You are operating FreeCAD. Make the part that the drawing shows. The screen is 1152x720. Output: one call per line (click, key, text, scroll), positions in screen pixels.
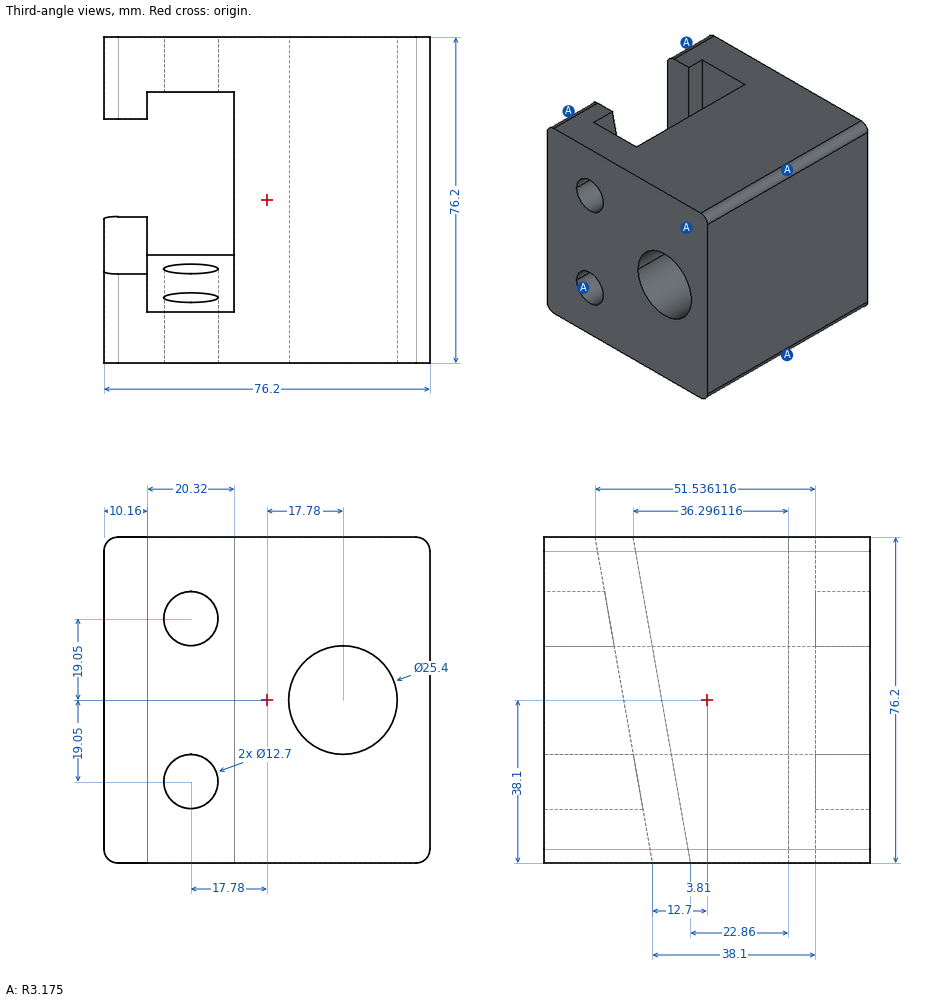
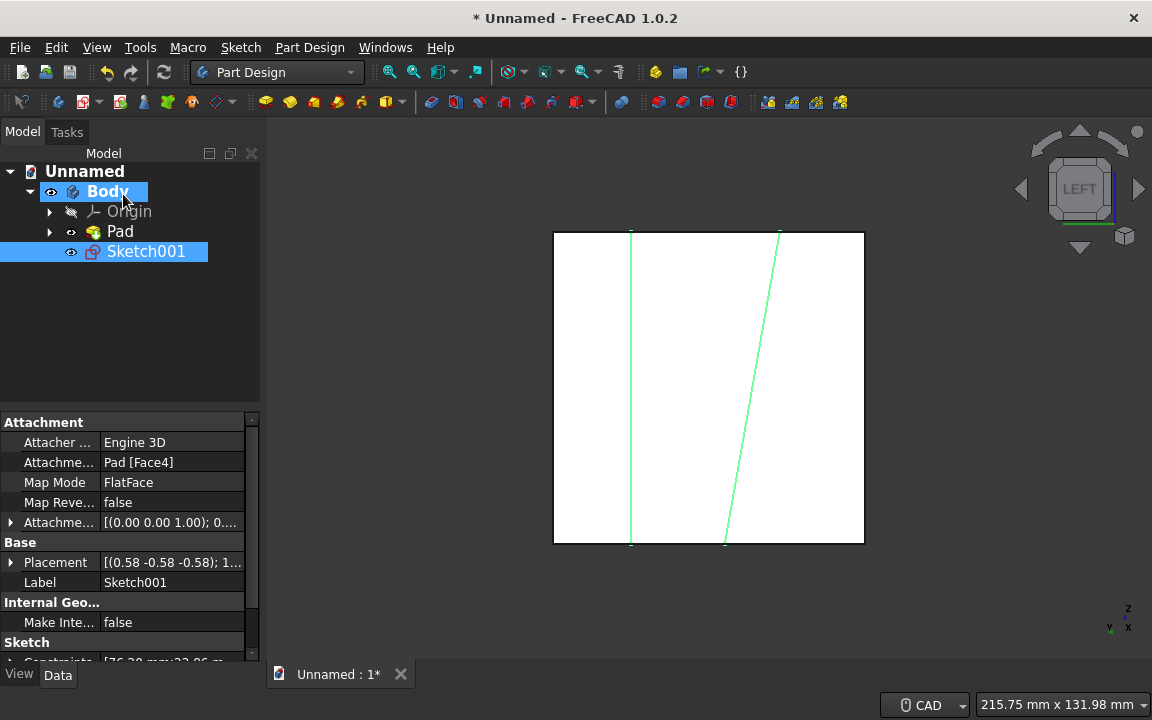
click(432, 102)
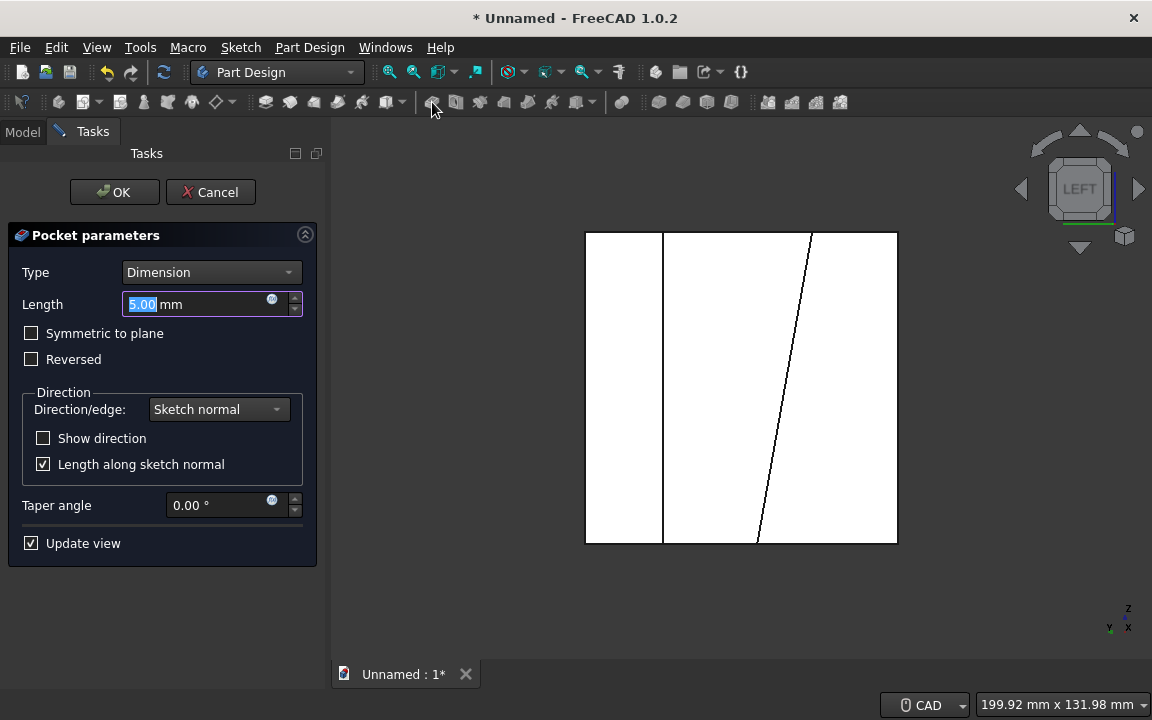
text(10.16)
key(Tab)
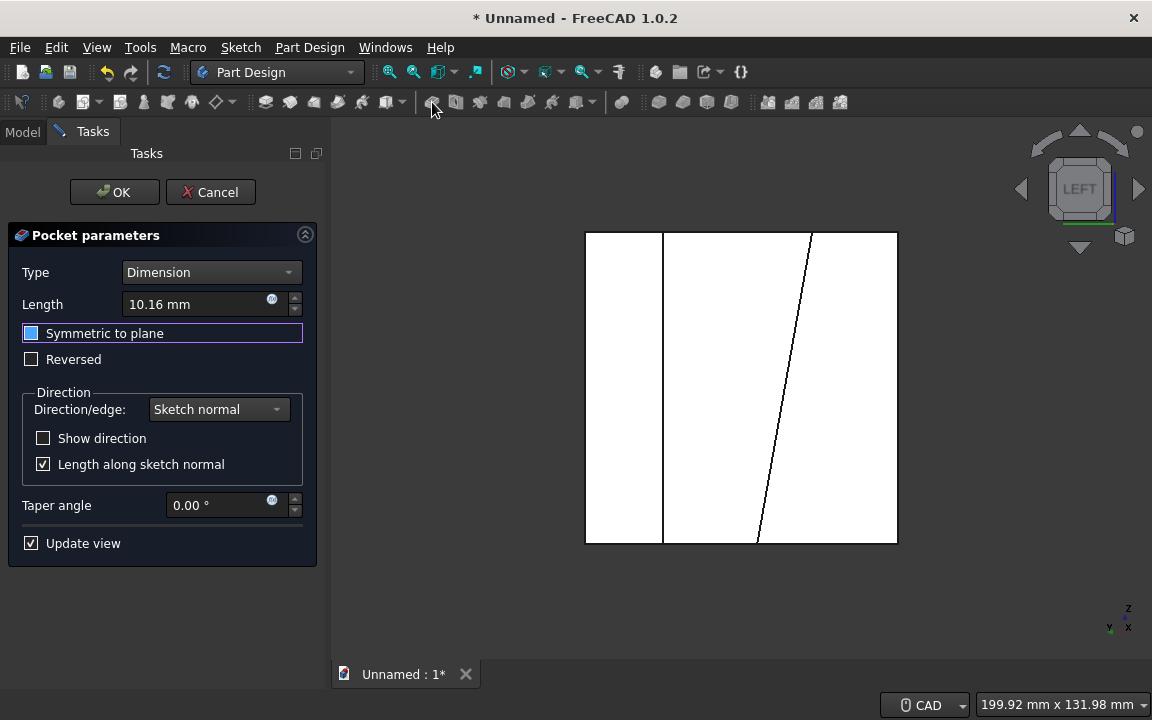
click(115, 192)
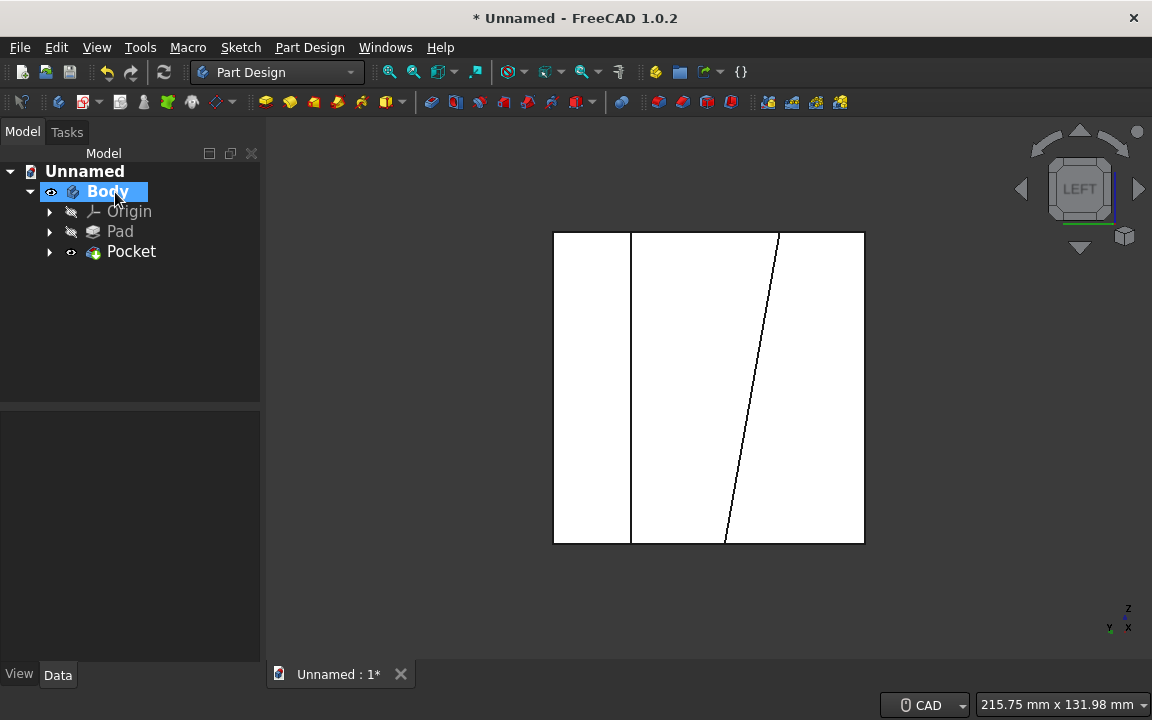
click(705, 298)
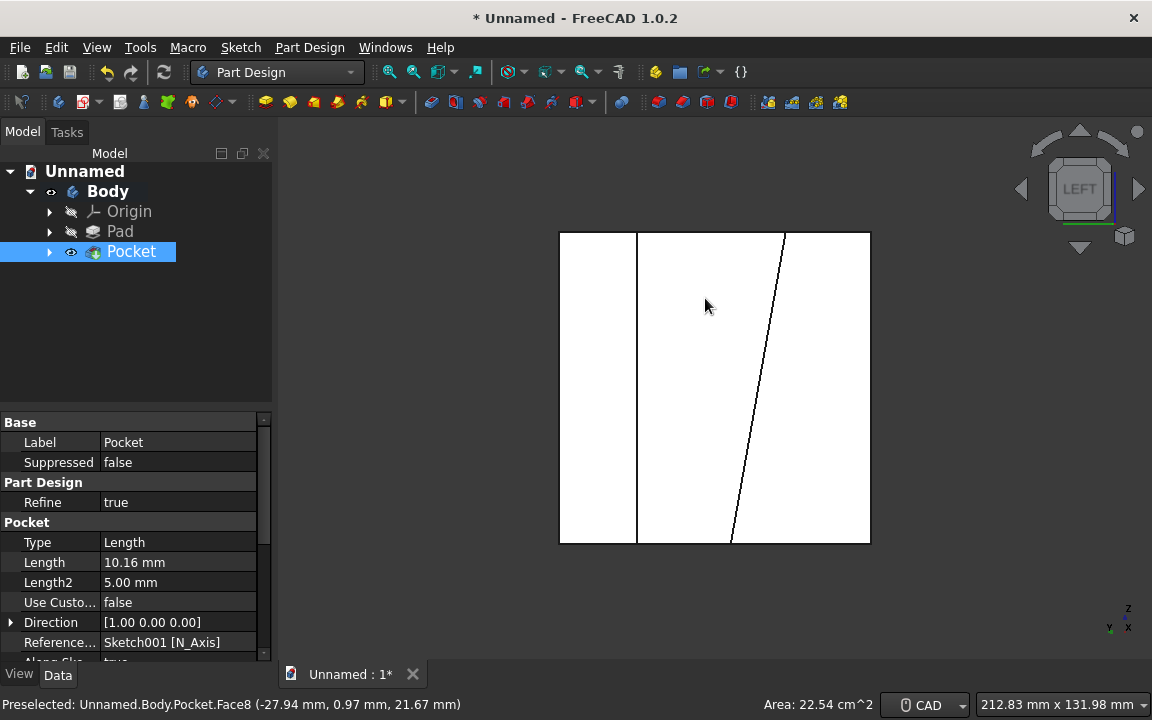
click(84, 102)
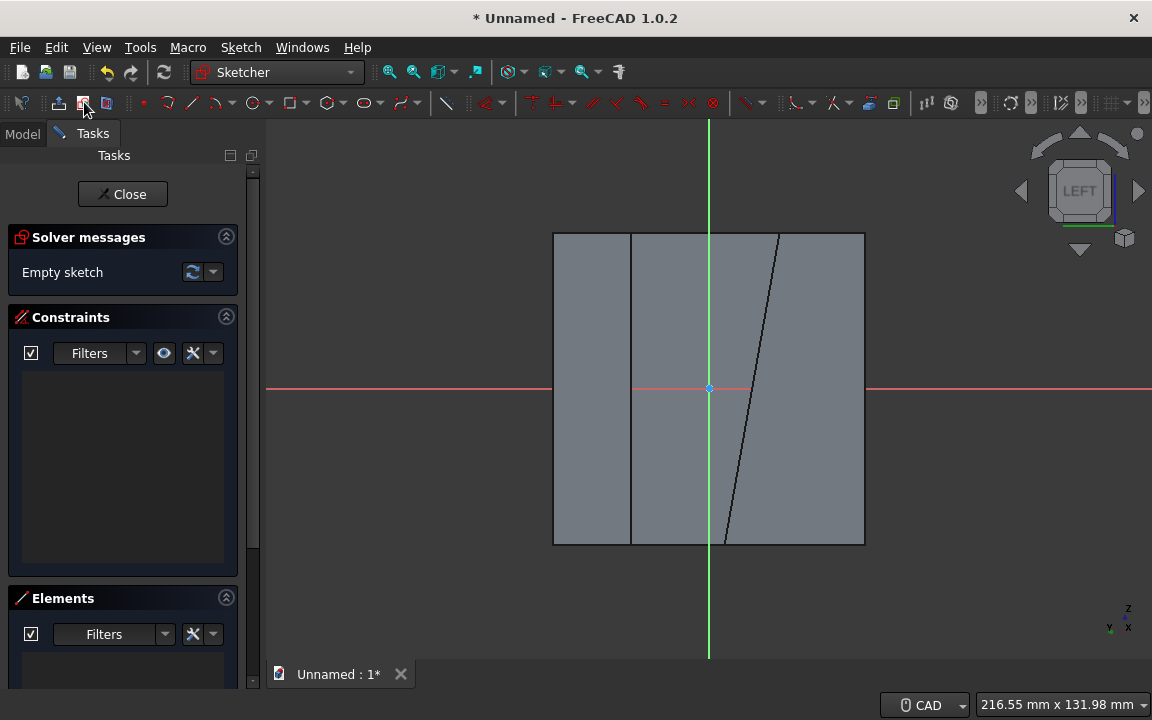
click(168, 104)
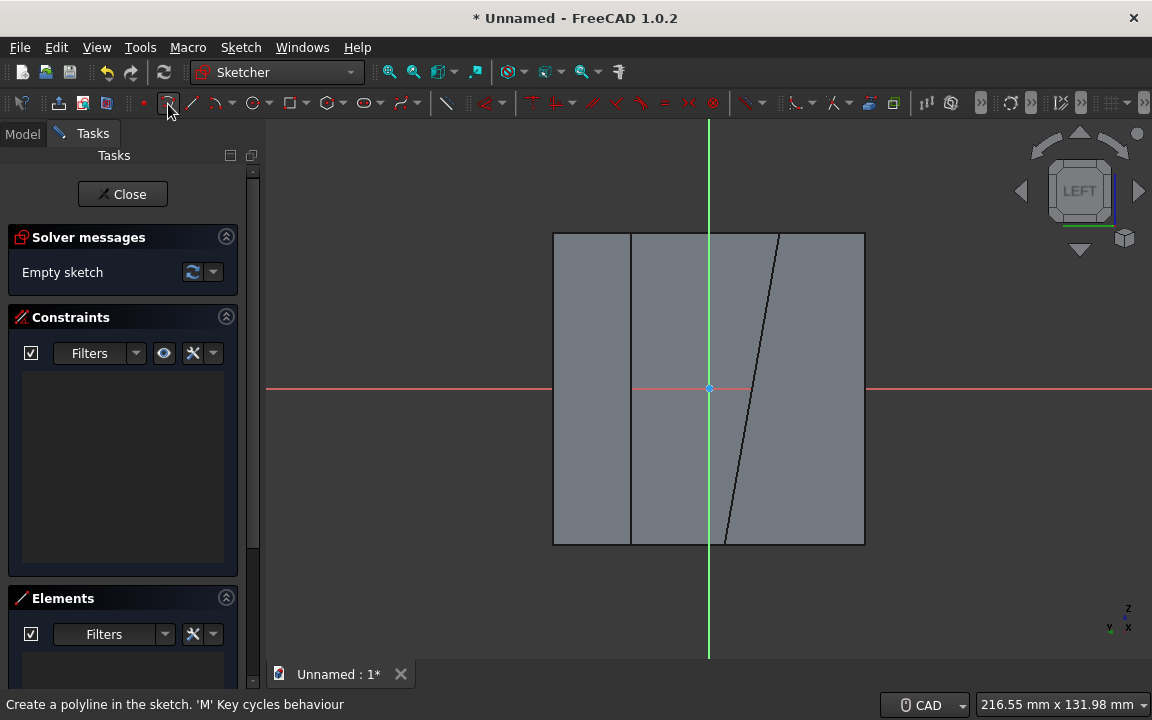
click(761, 545)
click(816, 233)
click(605, 233)
click(605, 545)
click(761, 546)
key(Escape)
key(Escape)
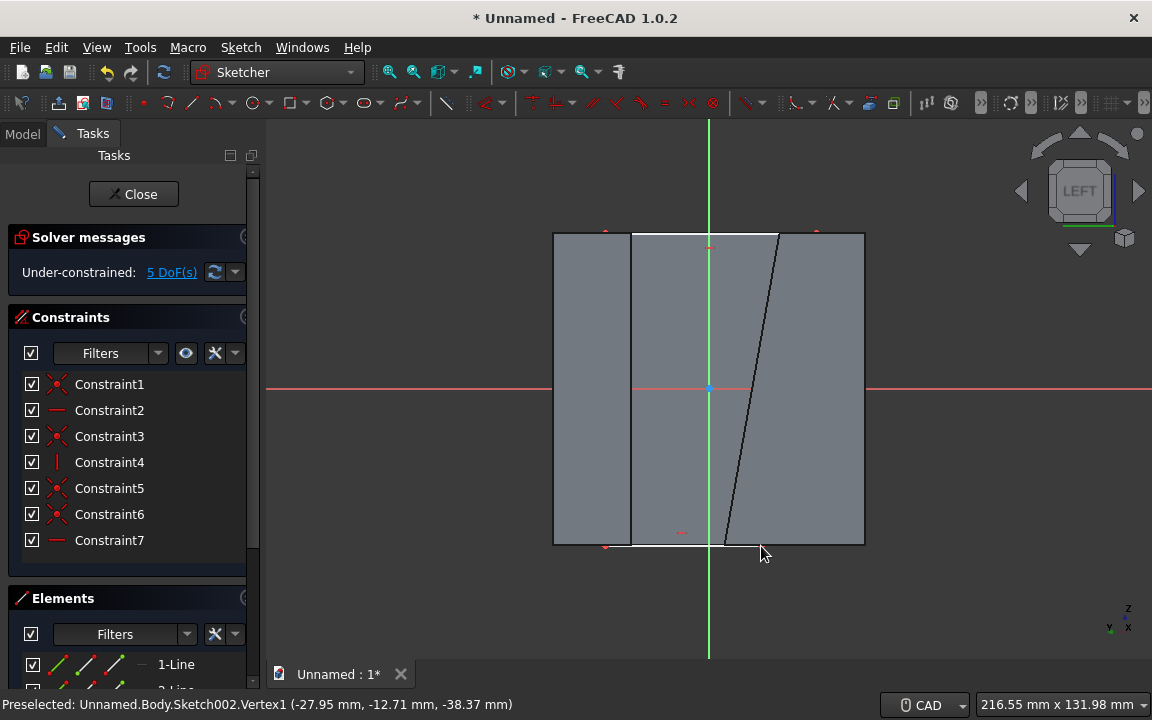
key(d)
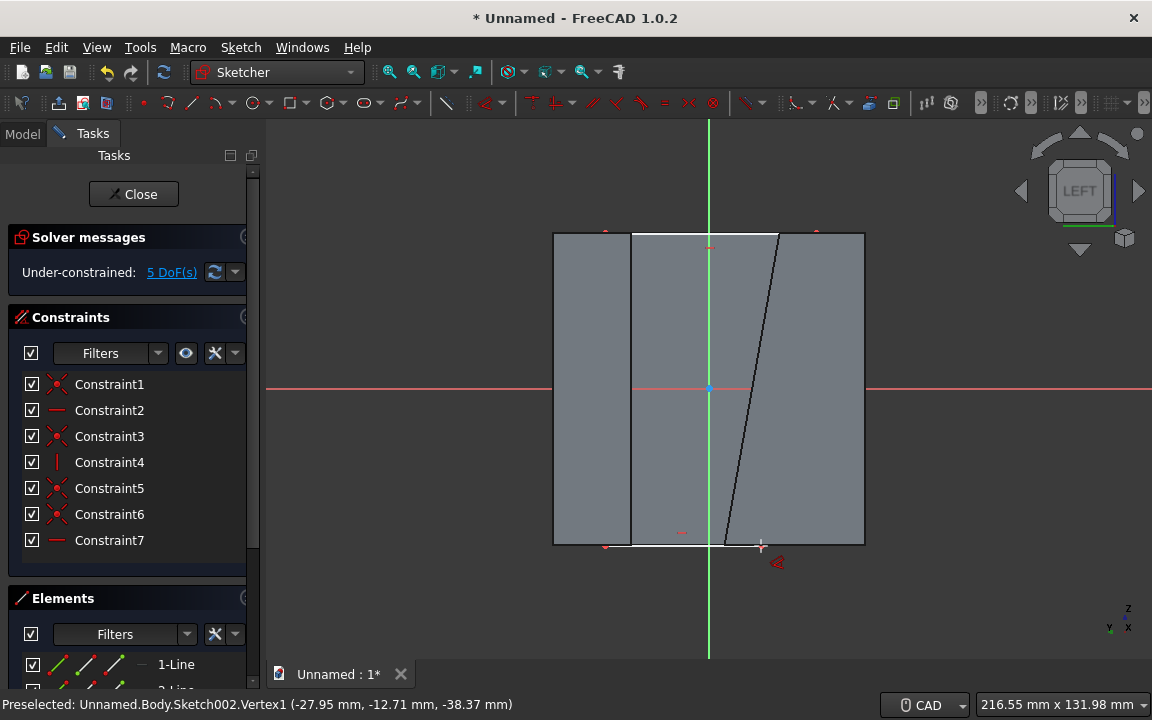
click(605, 328)
click(571, 318)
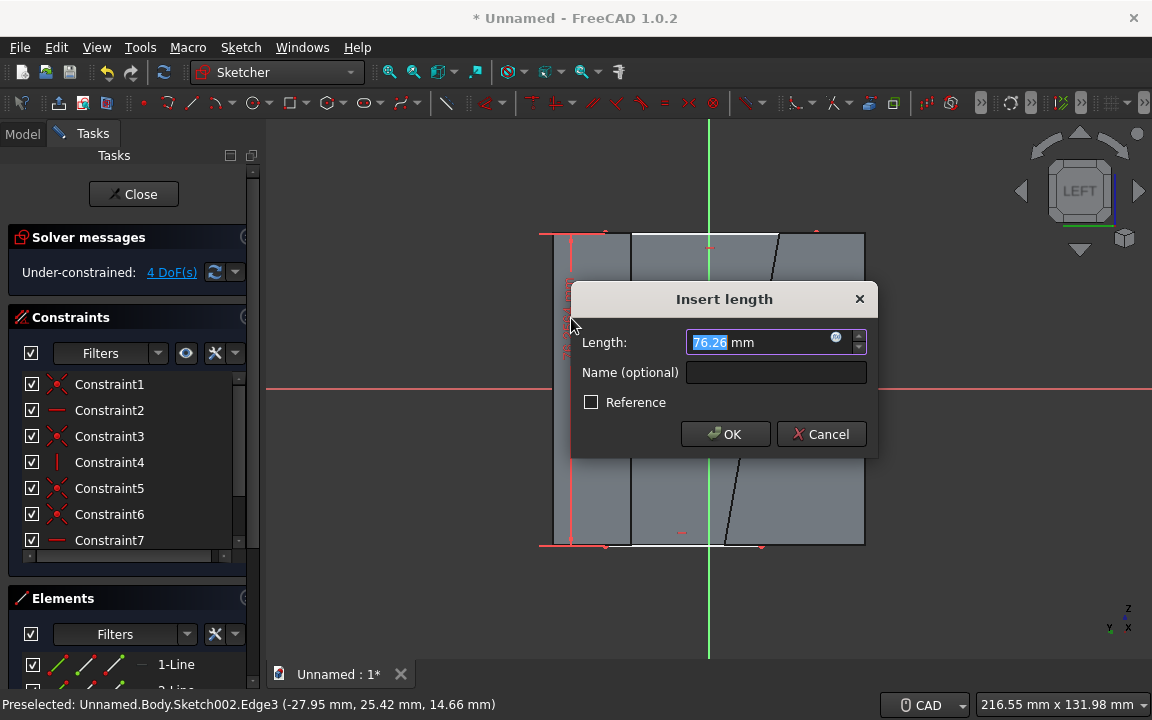
text(76.2)
key(Return)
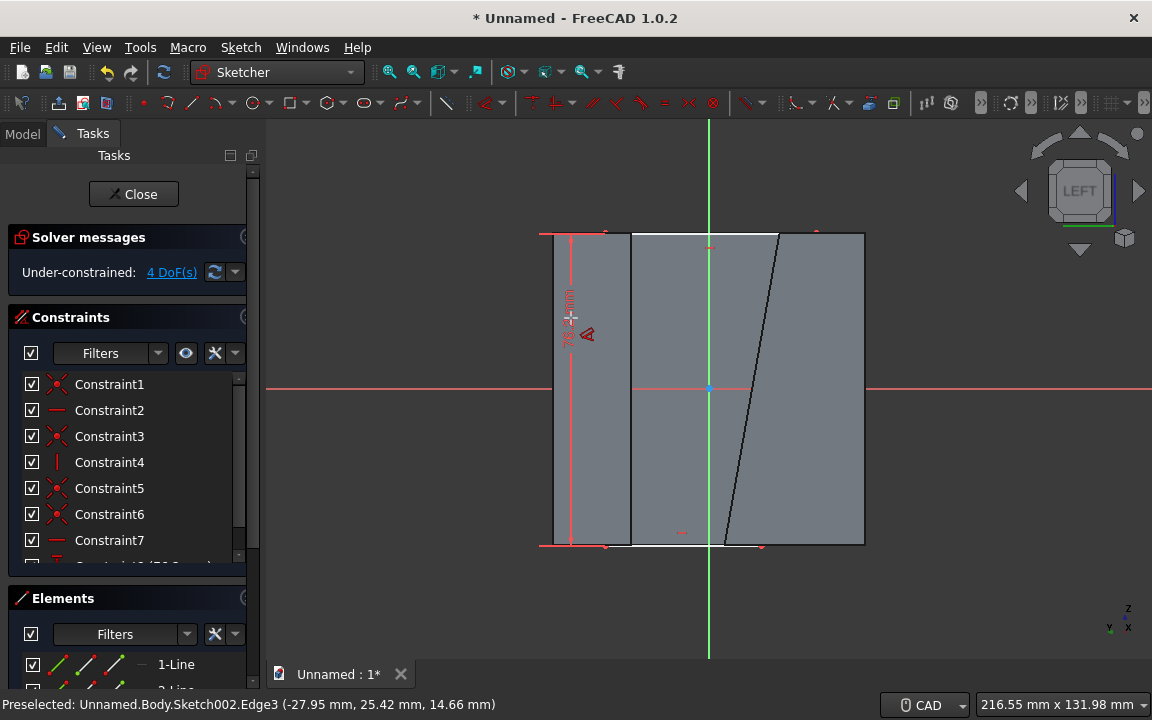
click(652, 546)
click(683, 580)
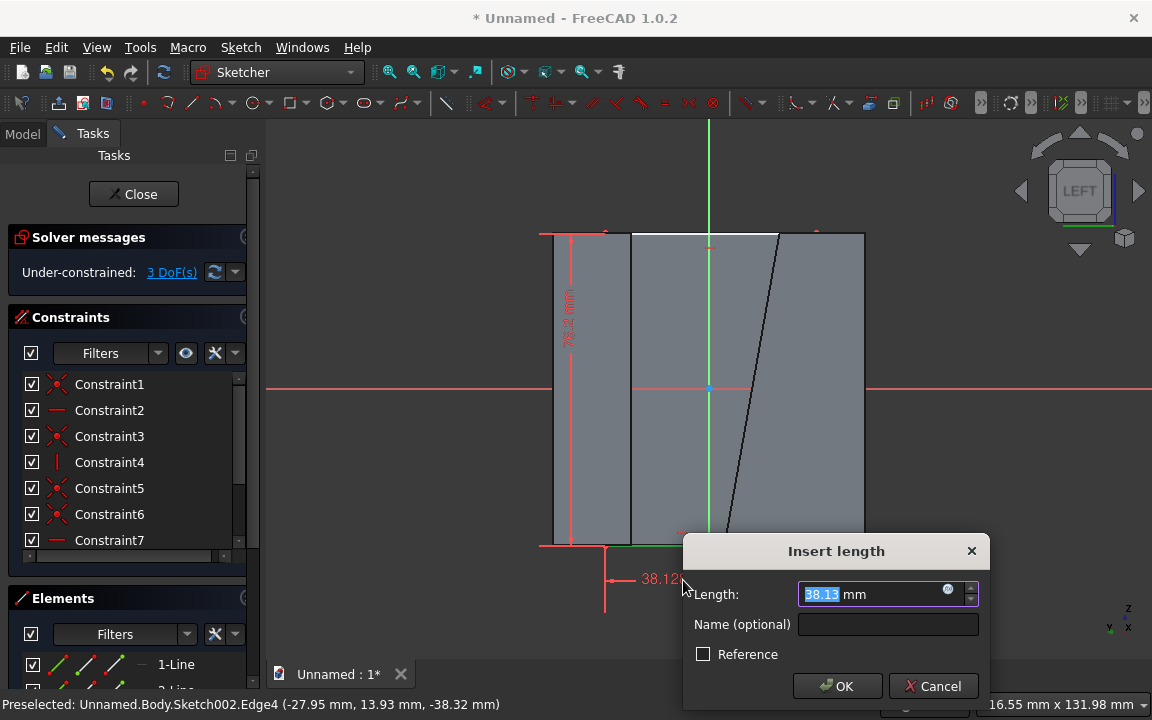
text(38.1)
key(Return)